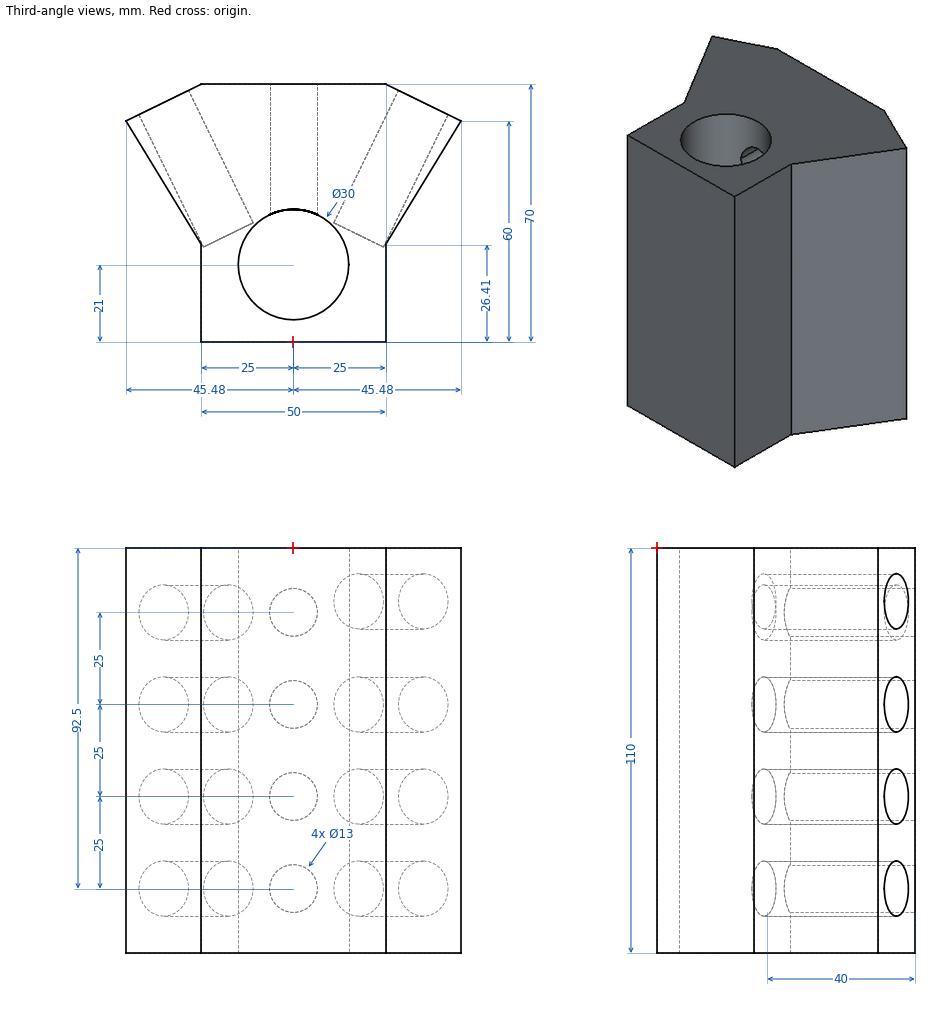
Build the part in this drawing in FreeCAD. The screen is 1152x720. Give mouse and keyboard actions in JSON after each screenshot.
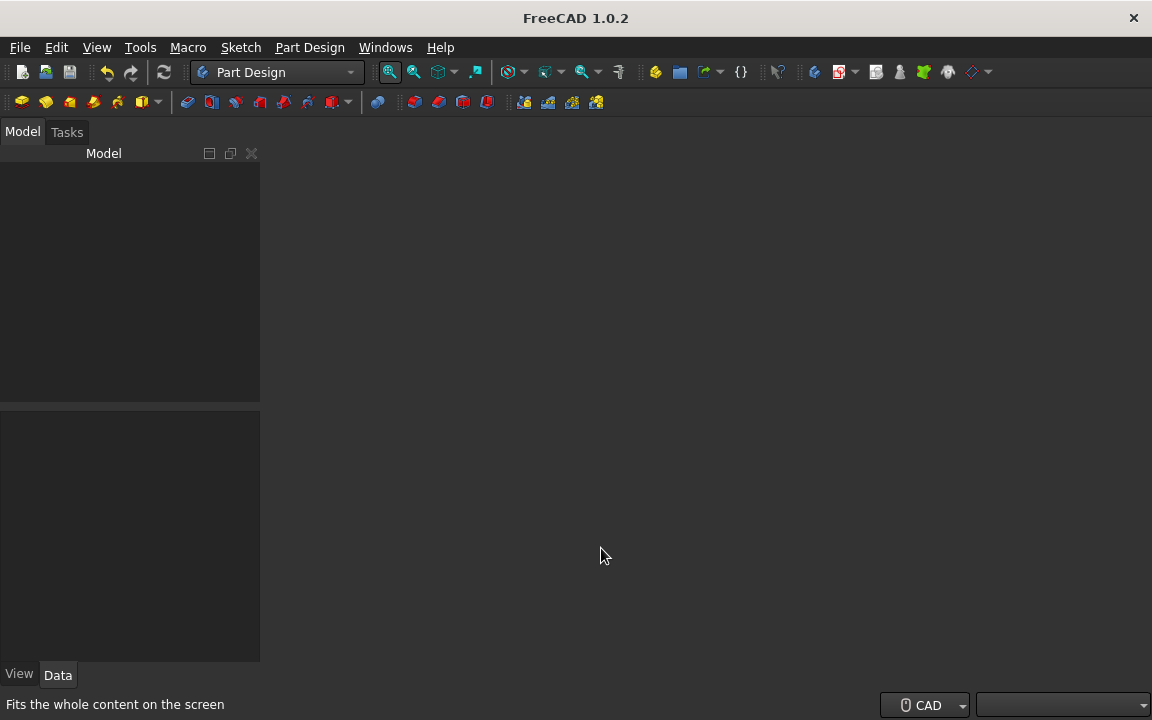
{"action": "left_click", "coordinate": [22, 72]}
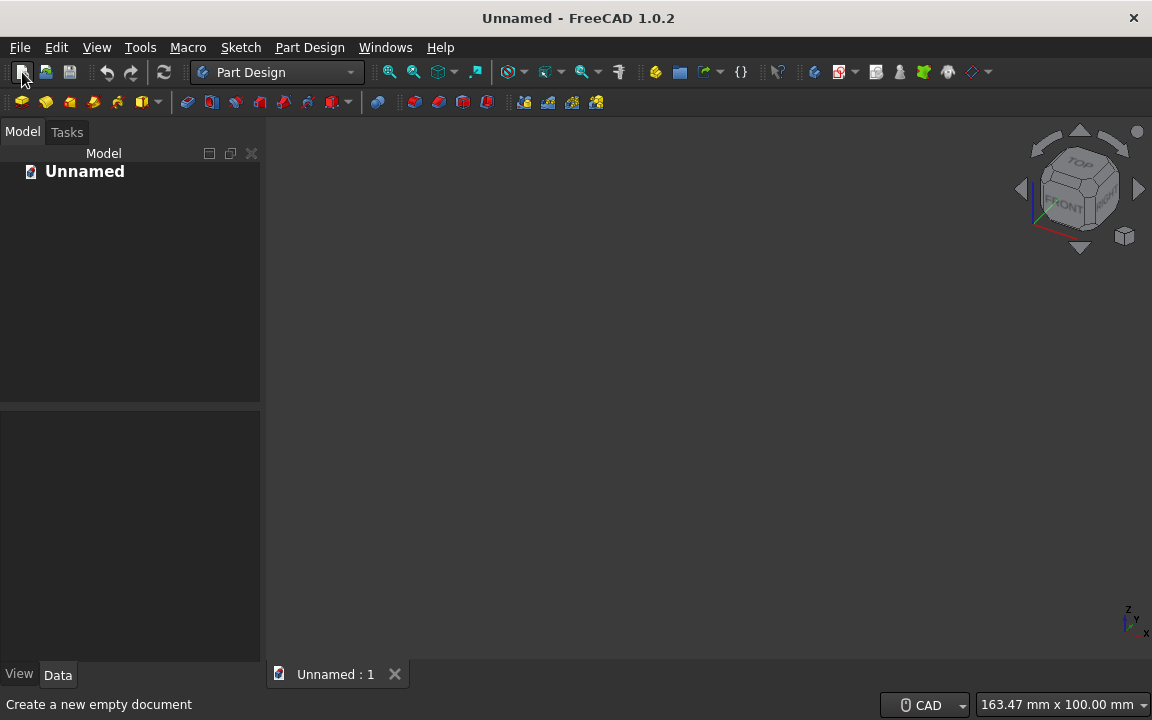
{"action": "left_click", "coordinate": [840, 72]}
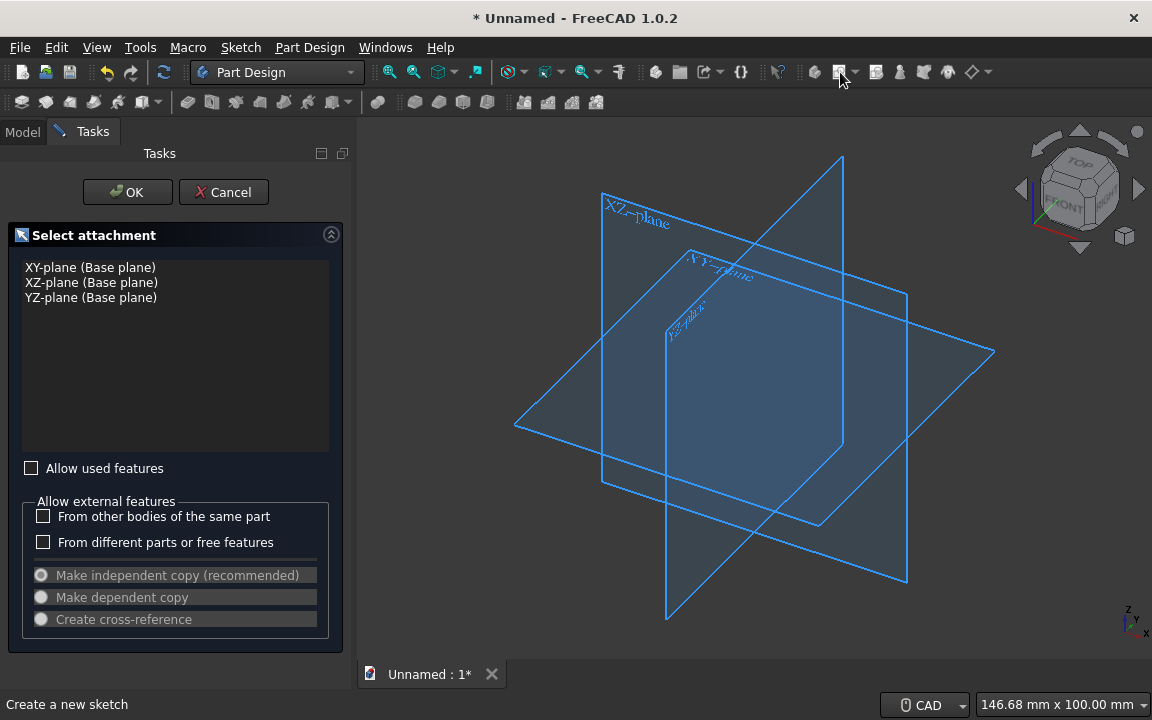
{"action": "left_click", "coordinate": [82, 268]}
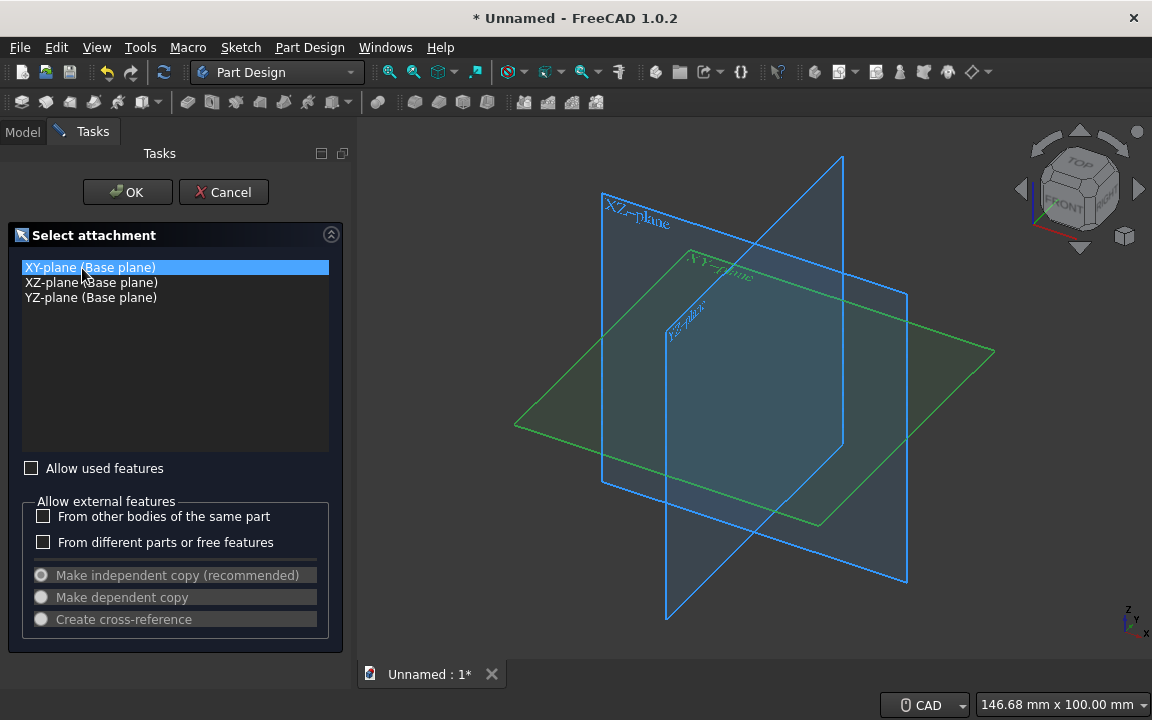
{"action": "left_click", "coordinate": [128, 192]}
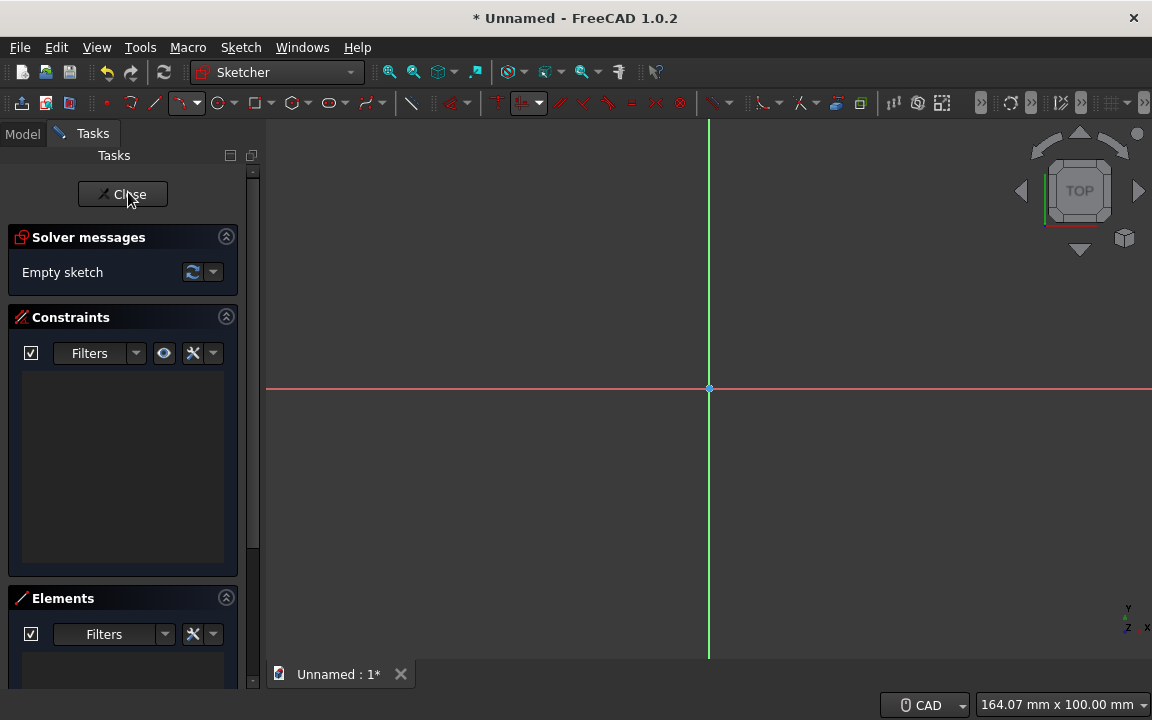
{"action": "scroll", "coordinate": [501, 631], "scroll_direction": "down", "scroll_amount": 2}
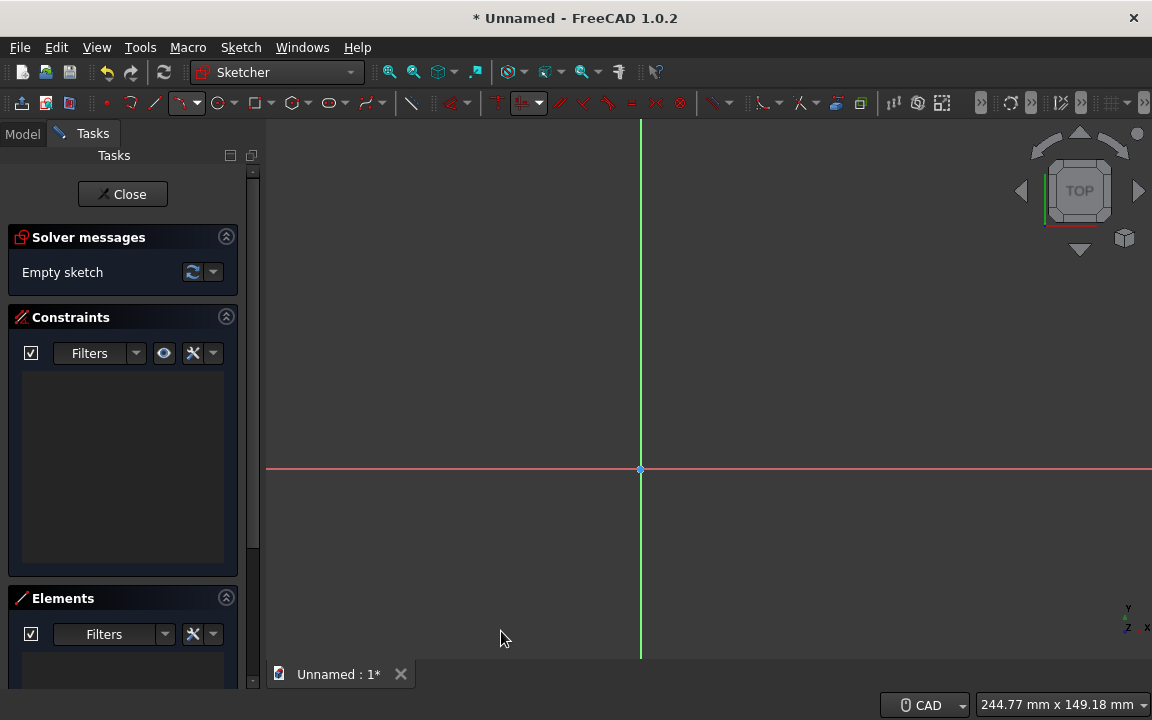
{"action": "key", "text": "g m"}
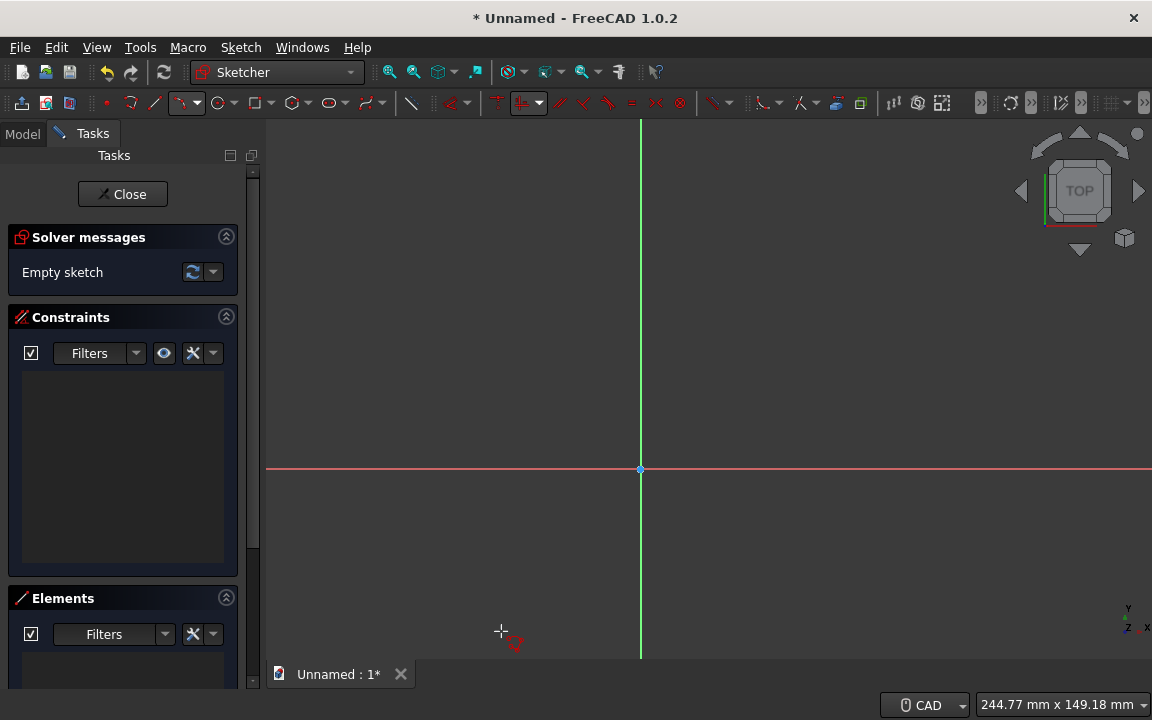
{"action": "left_click", "coordinate": [550, 469]}
{"action": "left_click", "coordinate": [731, 460]}
{"action": "left_click", "coordinate": [731, 373]}
{"action": "left_click", "coordinate": [805, 252]}
{"action": "left_click", "coordinate": [731, 216]}
{"action": "left_click", "coordinate": [550, 216]}
{"action": "left_click", "coordinate": [476, 252]}
{"action": "left_click", "coordinate": [550, 373]}
{"action": "left_click", "coordinate": [550, 469]}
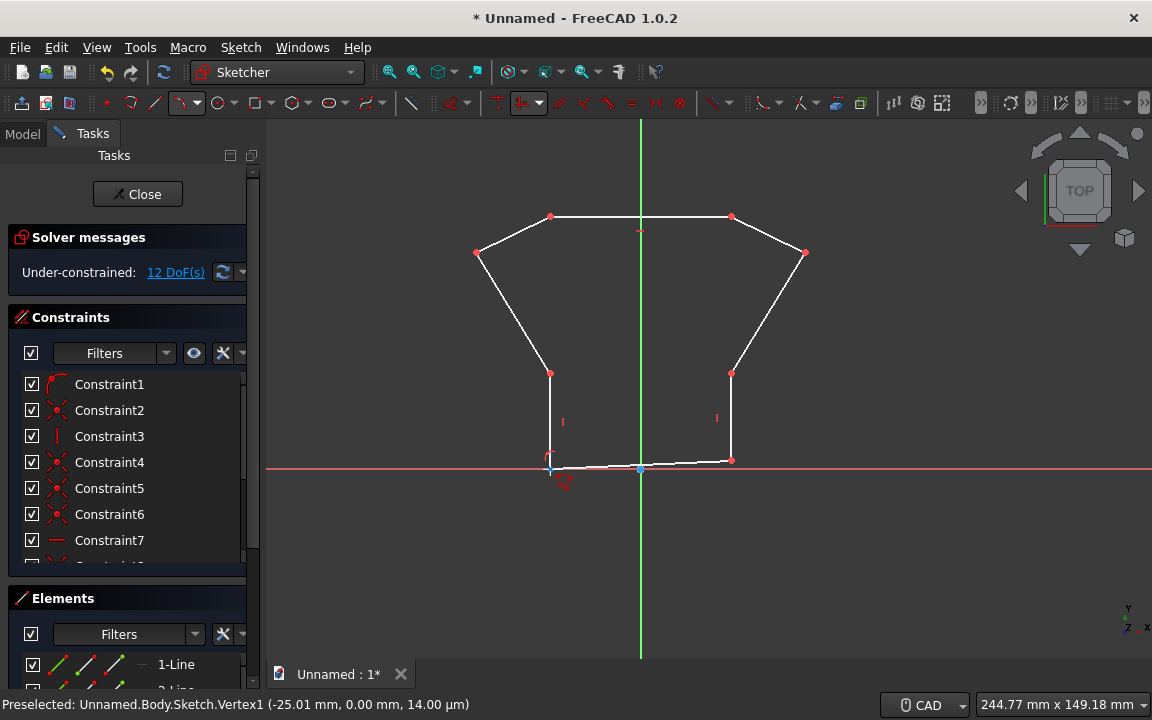
{"action": "left_click", "coordinate": [218, 104]}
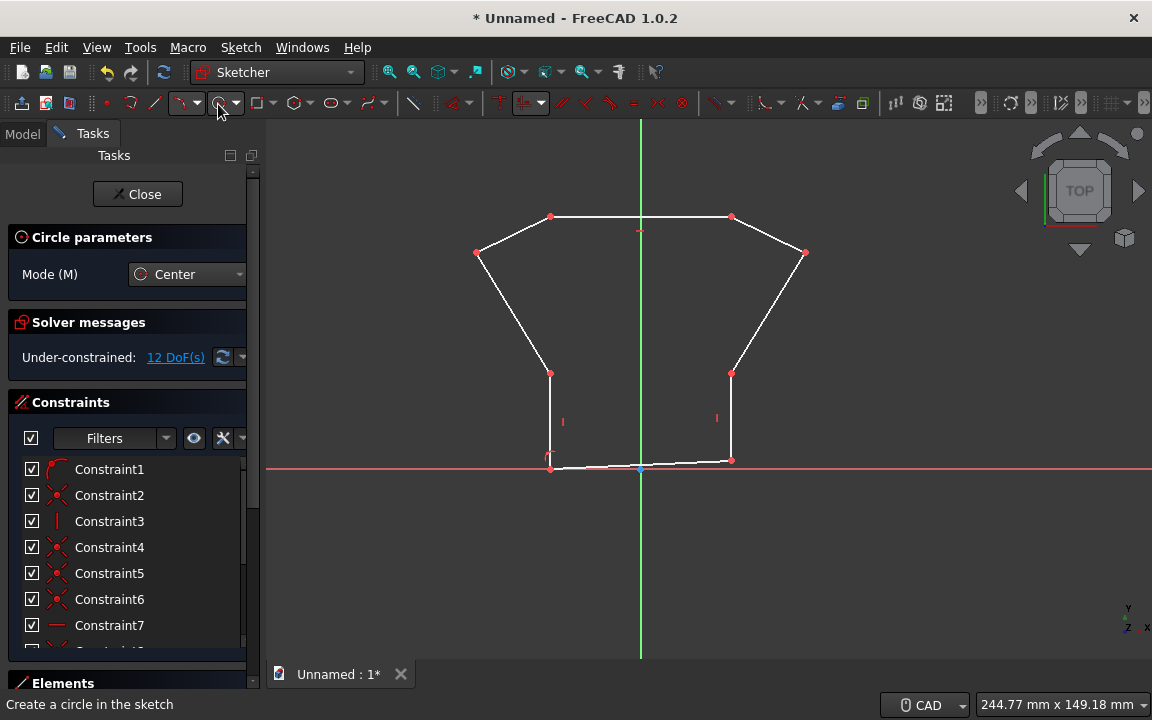
{"action": "left_click", "coordinate": [641, 393]}
{"action": "left_click", "coordinate": [679, 355]}
{"action": "key", "text": "Escape"}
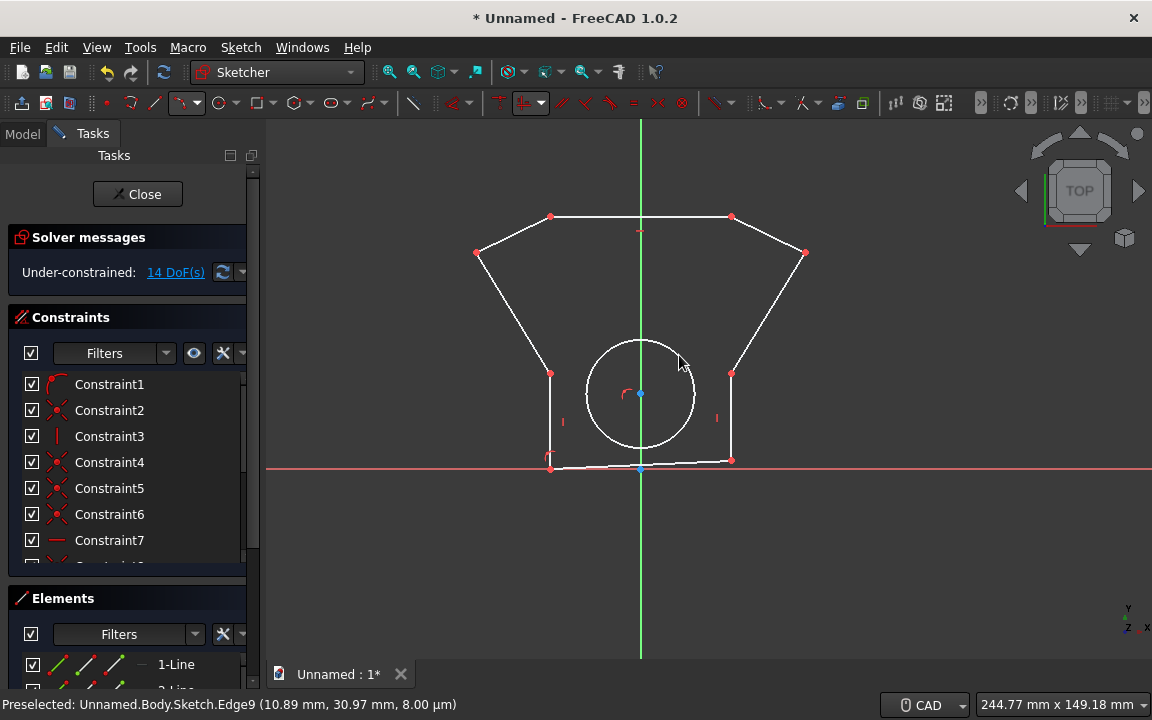
{"action": "left_click", "coordinate": [604, 467]}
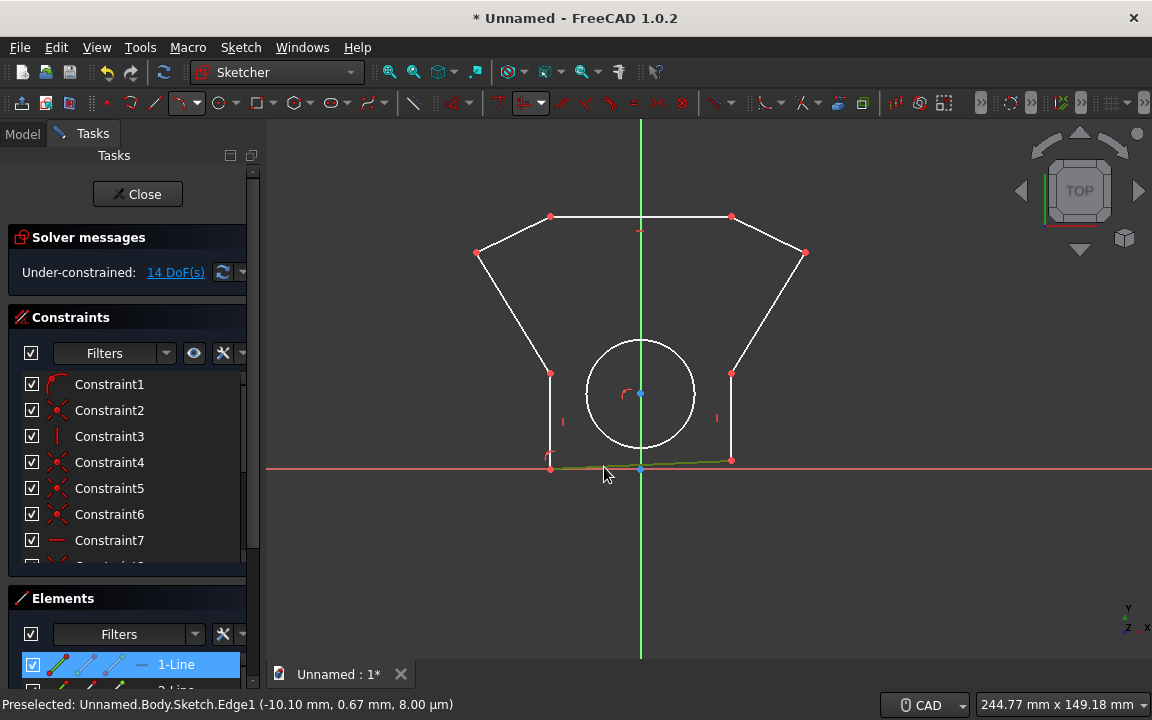
{"action": "left_click", "coordinate": [544, 104]}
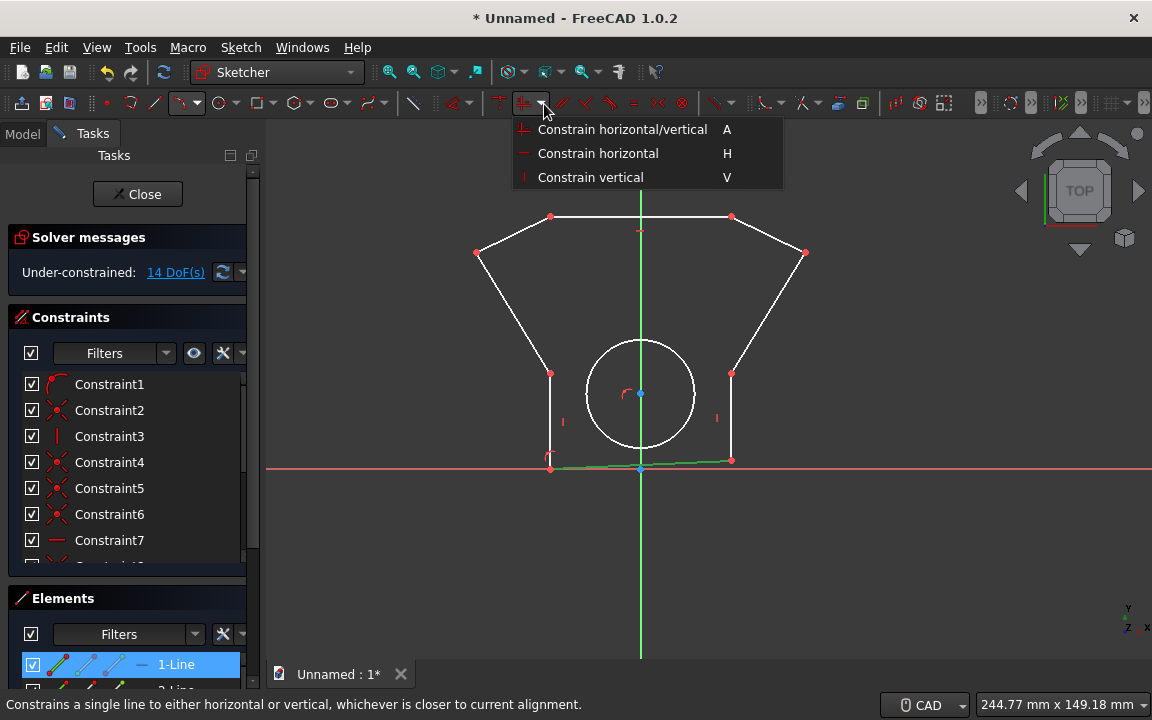
{"action": "left_click", "coordinate": [648, 153]}